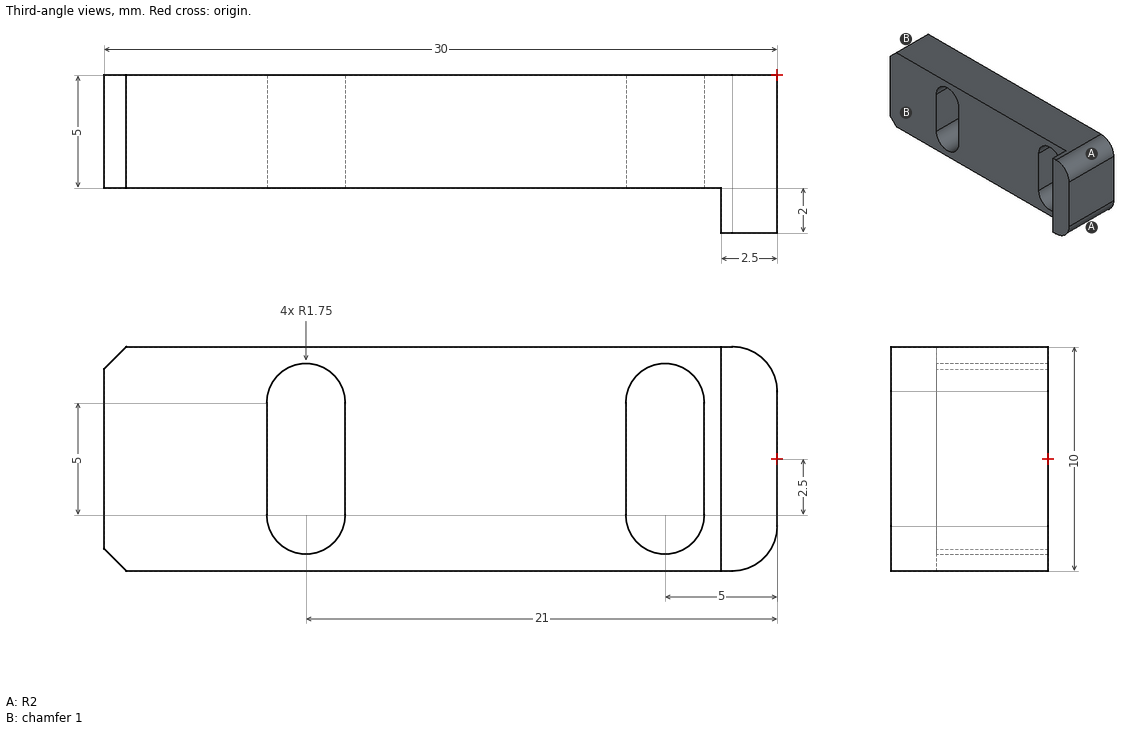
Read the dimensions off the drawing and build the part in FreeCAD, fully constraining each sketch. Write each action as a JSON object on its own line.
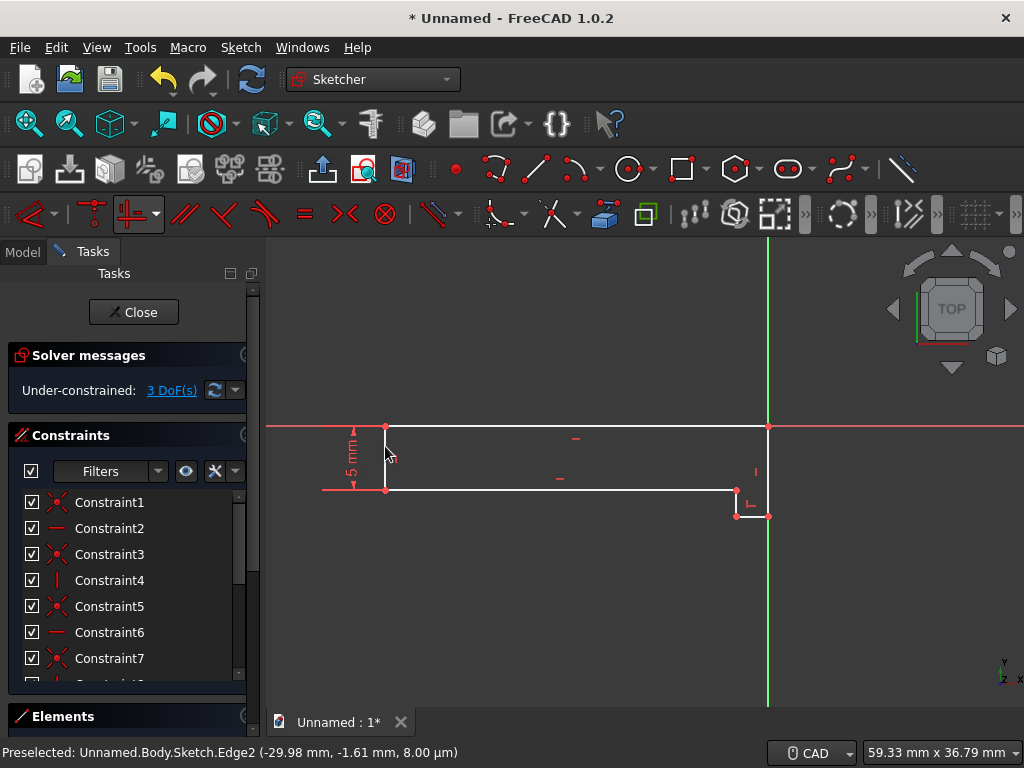
{"action": "scroll", "coordinate": [736, 501], "scroll_direction": "up", "scroll_amount": 3}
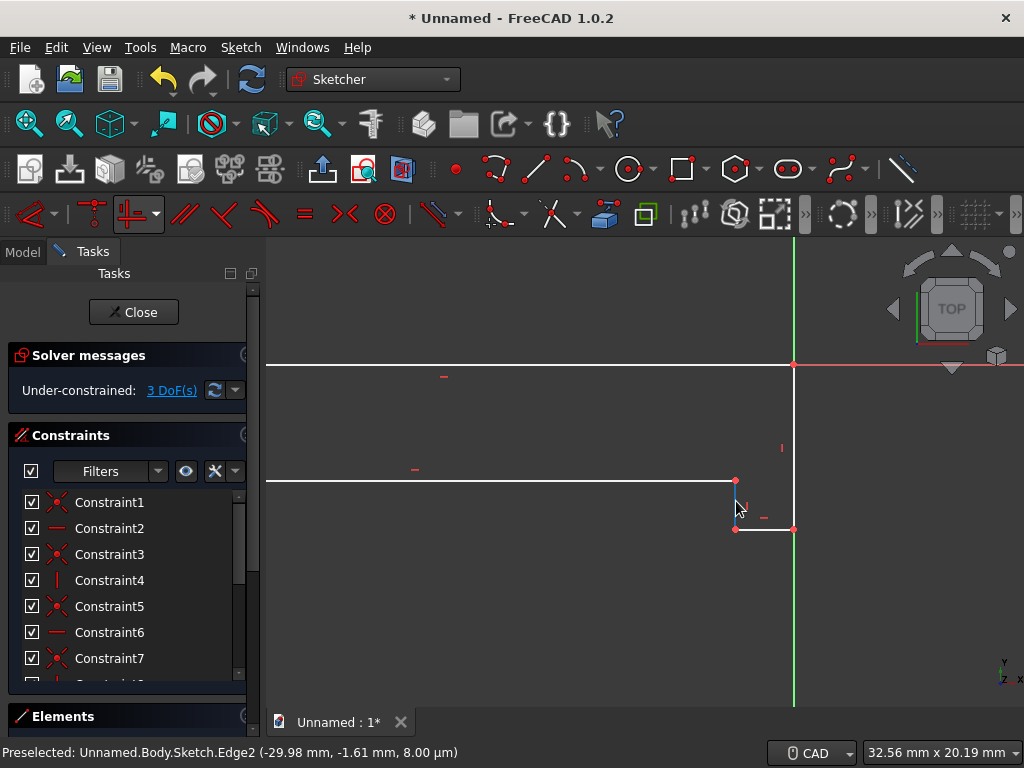
{"action": "left_click", "coordinate": [735, 500]}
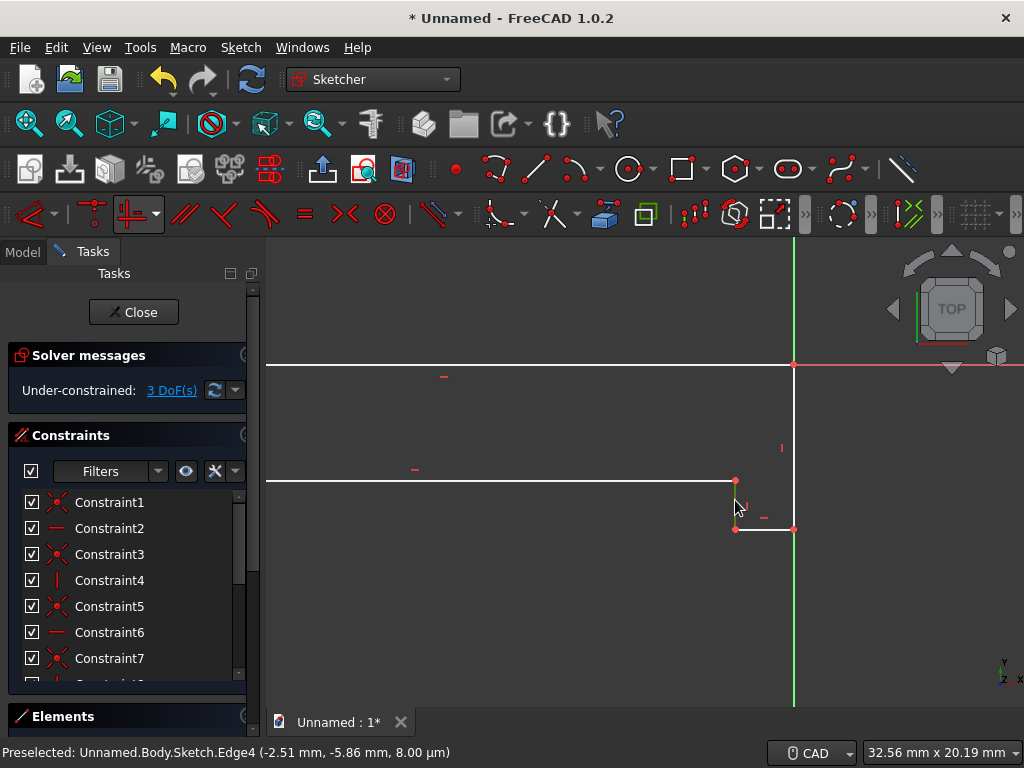
{"action": "key", "text": "i"}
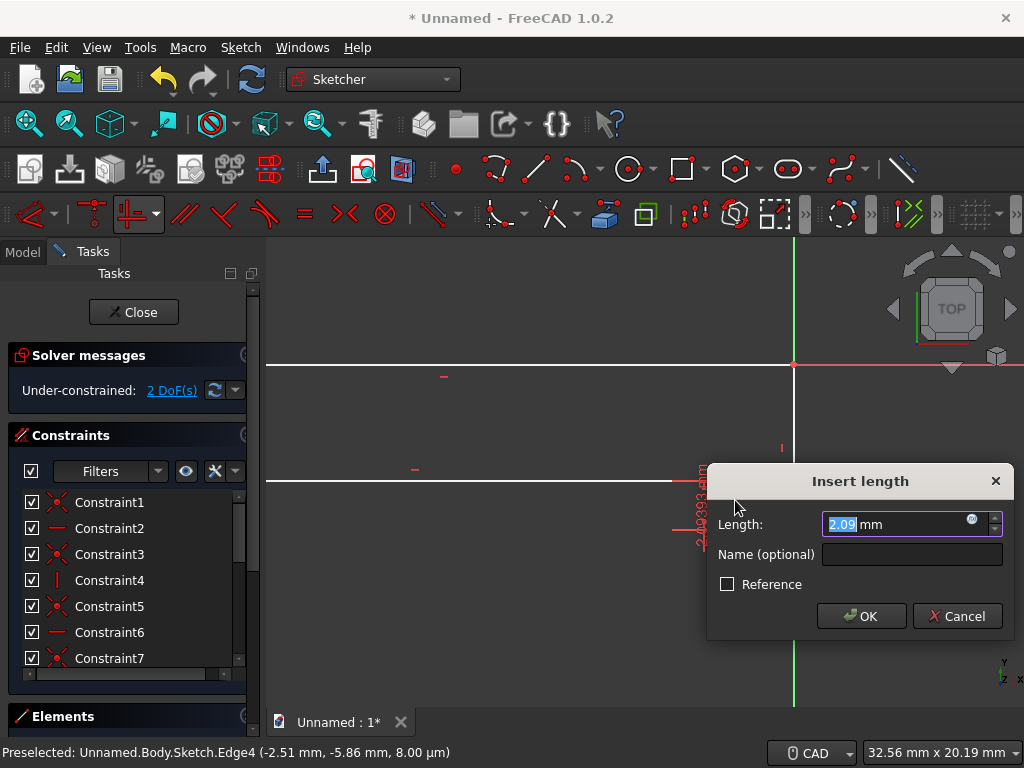
{"action": "type", "text": "2"}
{"action": "key", "text": "Return"}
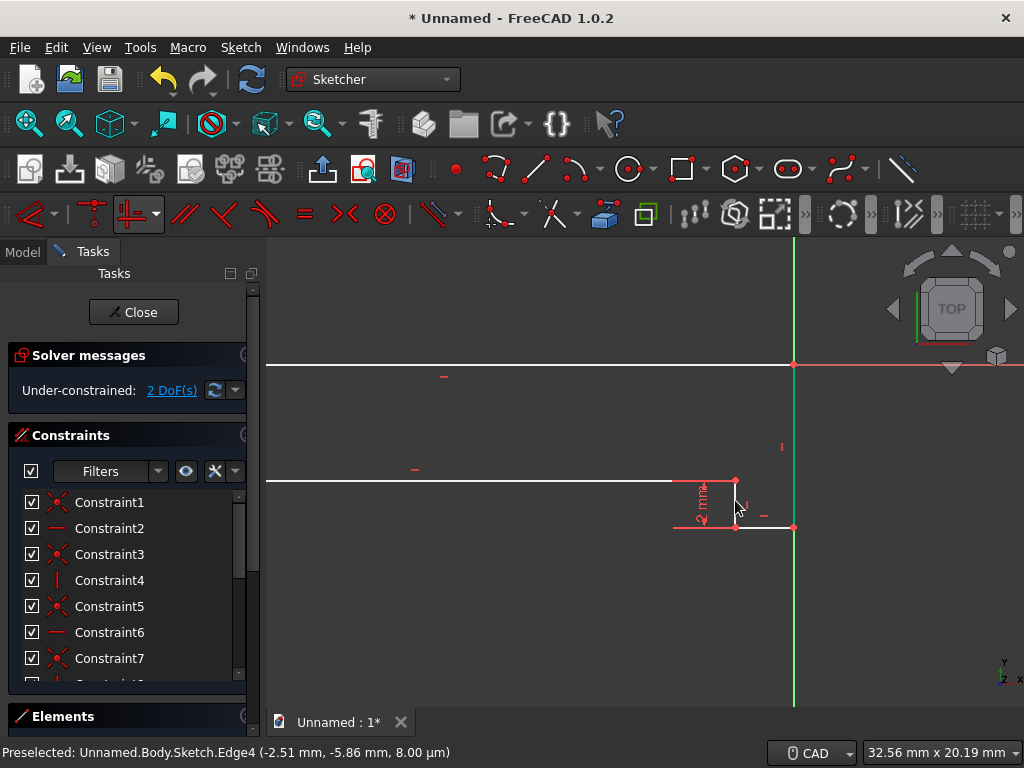
{"action": "left_click", "coordinate": [584, 365]}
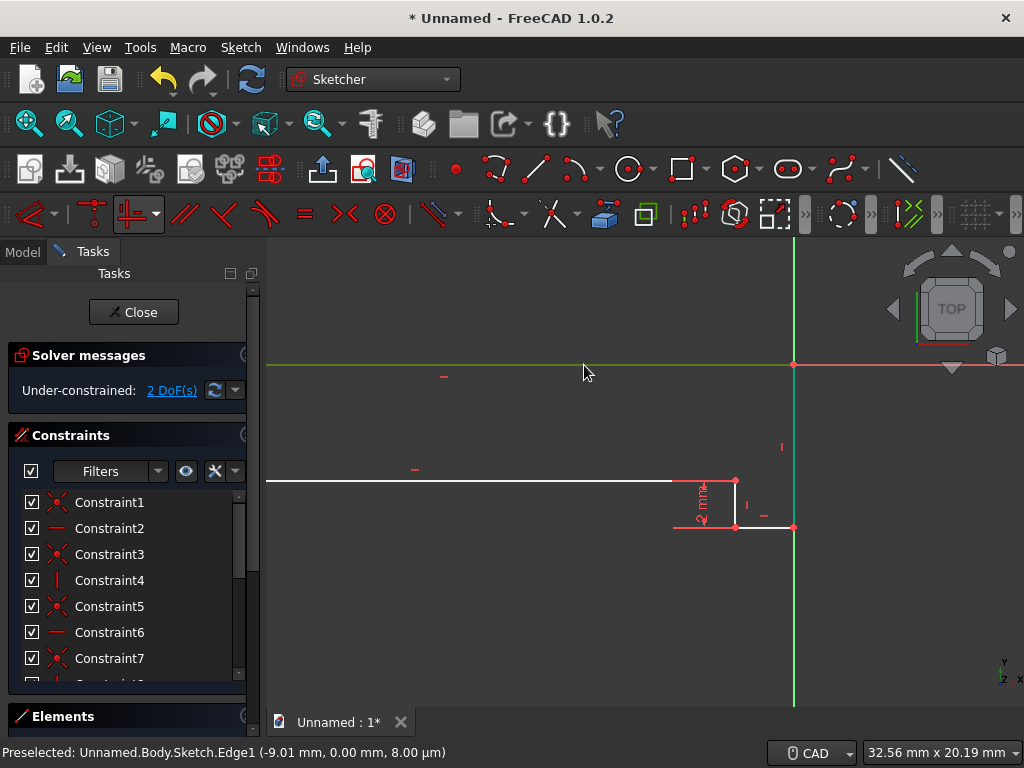
{"action": "key", "text": "l"}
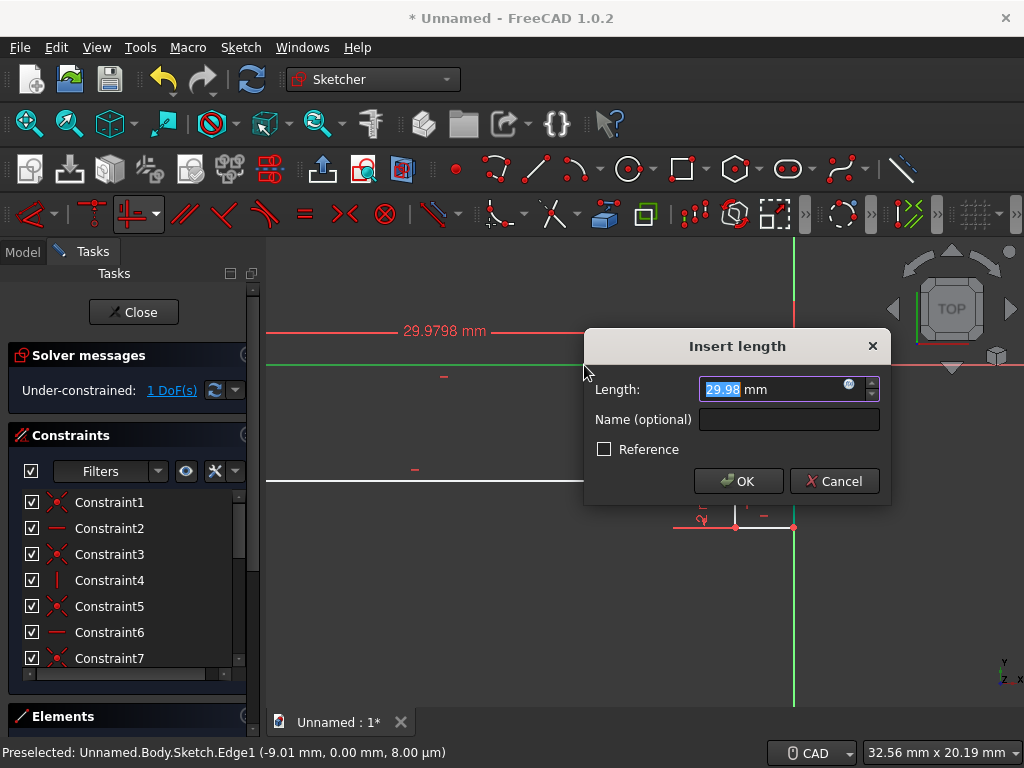
{"action": "type", "text": "30"}
{"action": "key", "text": "Return"}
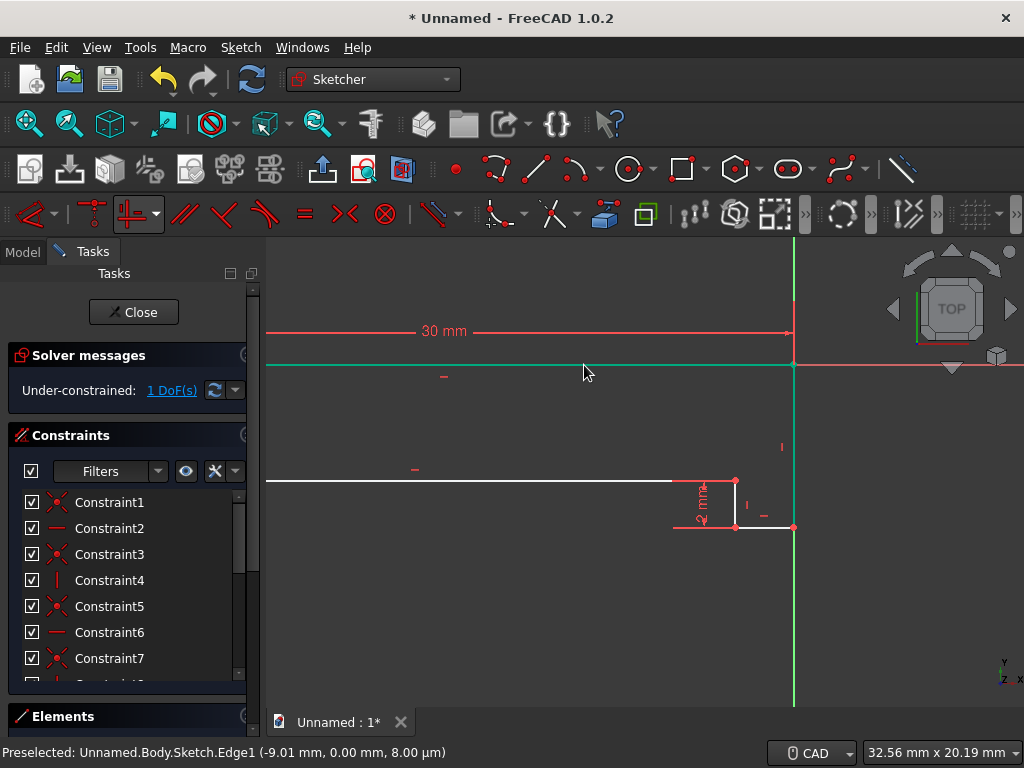
{"action": "left_click", "coordinate": [753, 528]}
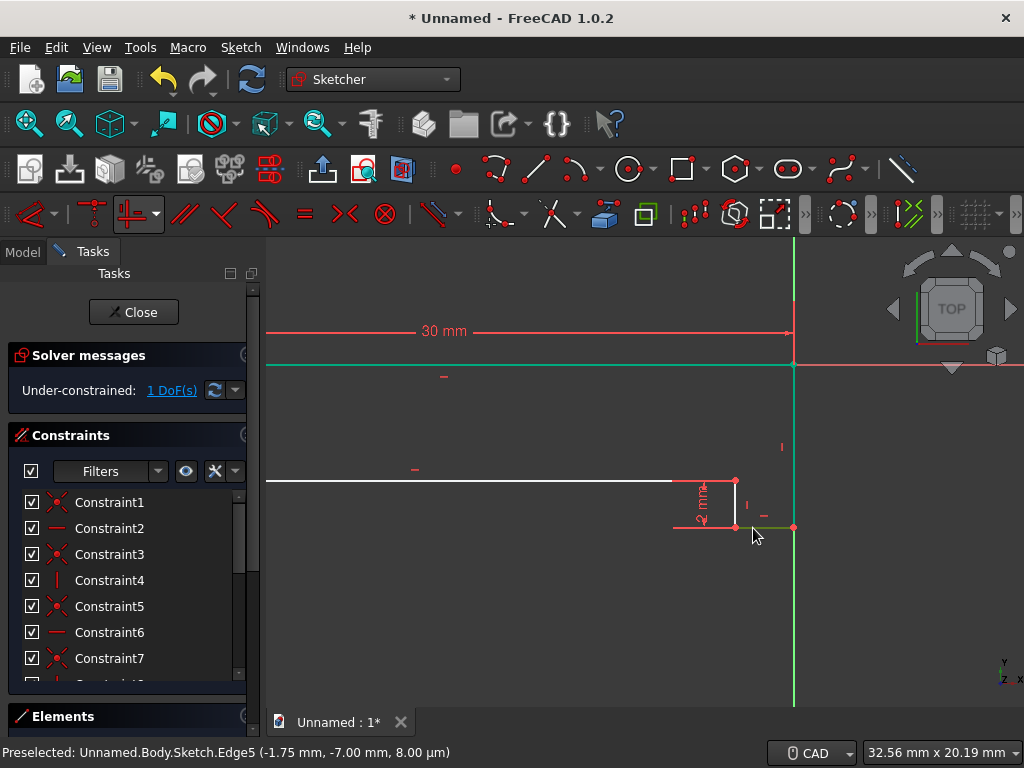
{"action": "key", "text": "l"}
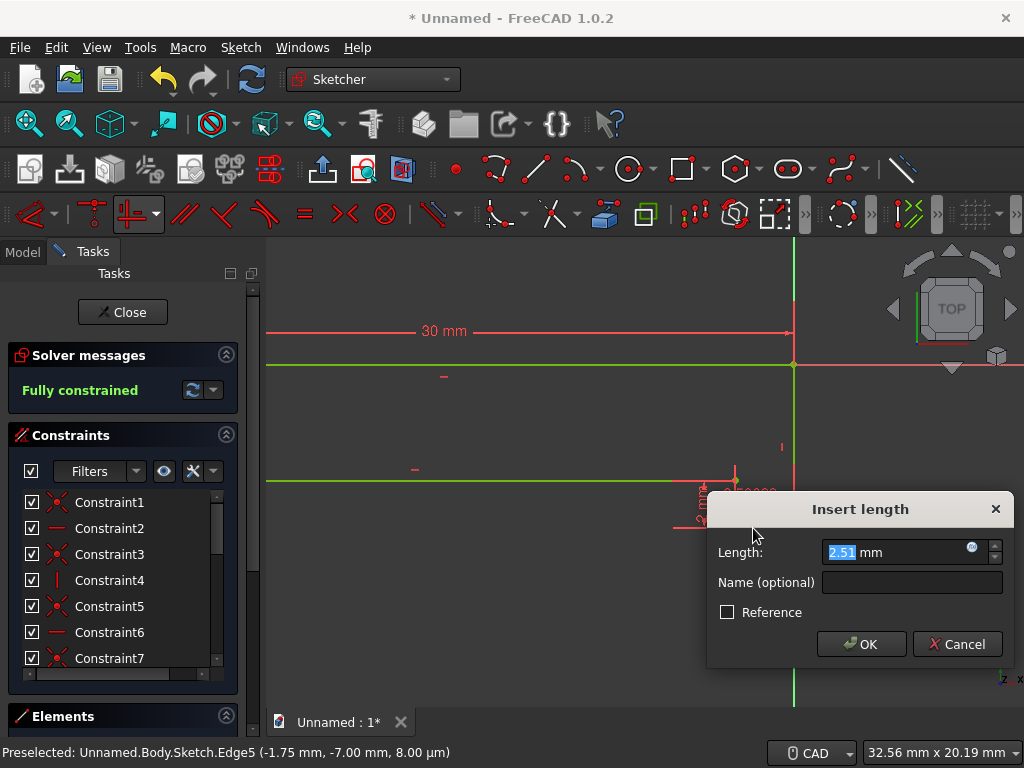
{"action": "type", "text": "2.5"}
{"action": "key", "text": "Return"}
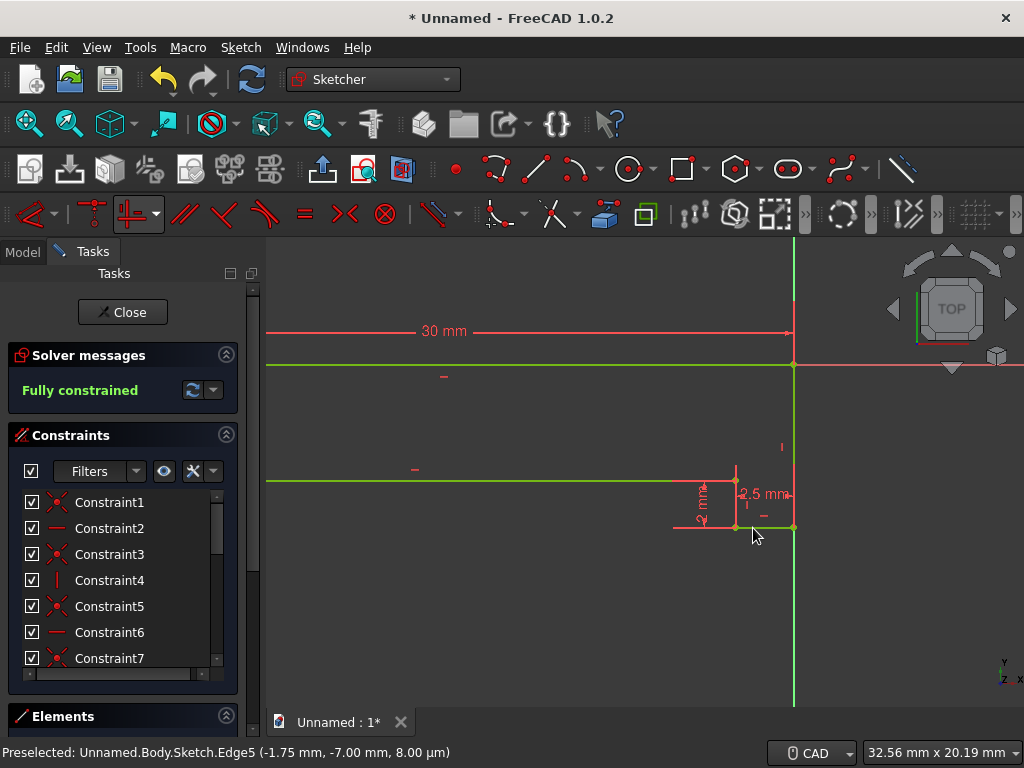
{"action": "left_click", "coordinate": [123, 312]}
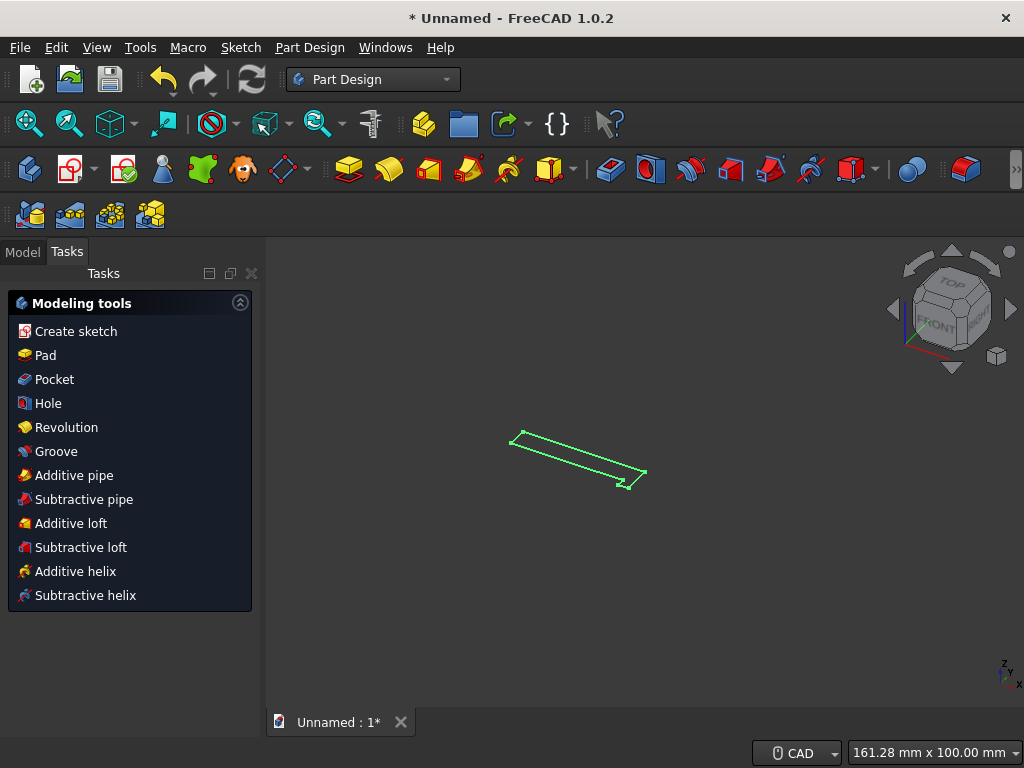
{"action": "left_click", "coordinate": [350, 170]}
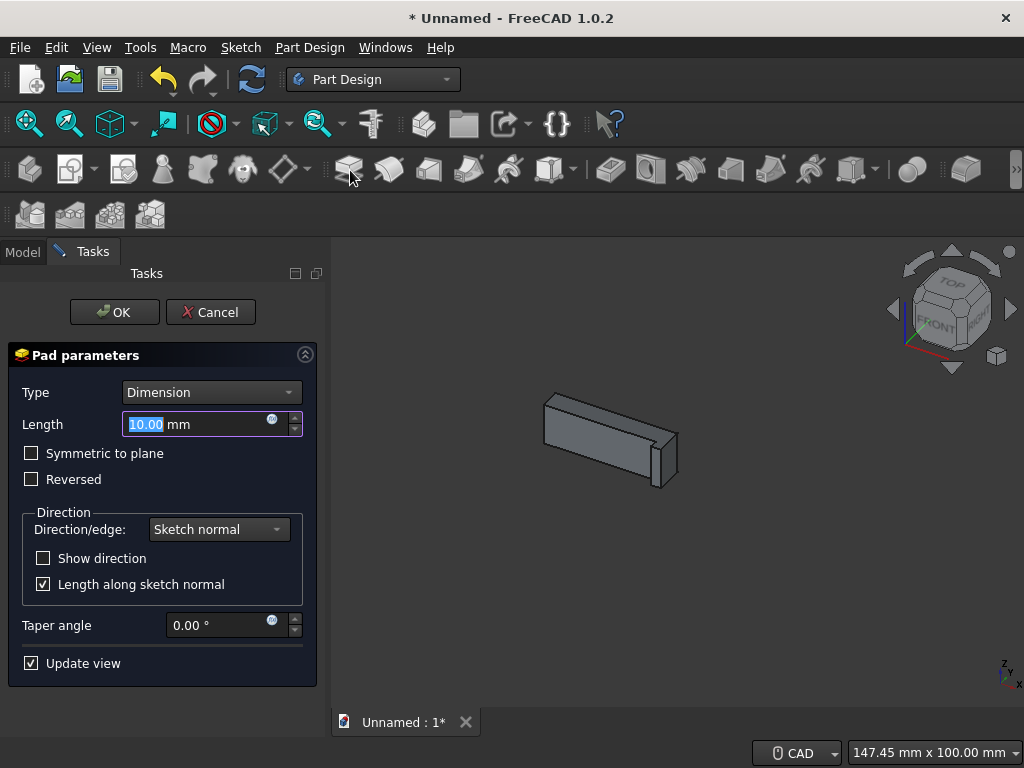
{"action": "type", "text": "10"}
{"action": "key", "text": "Tab"}